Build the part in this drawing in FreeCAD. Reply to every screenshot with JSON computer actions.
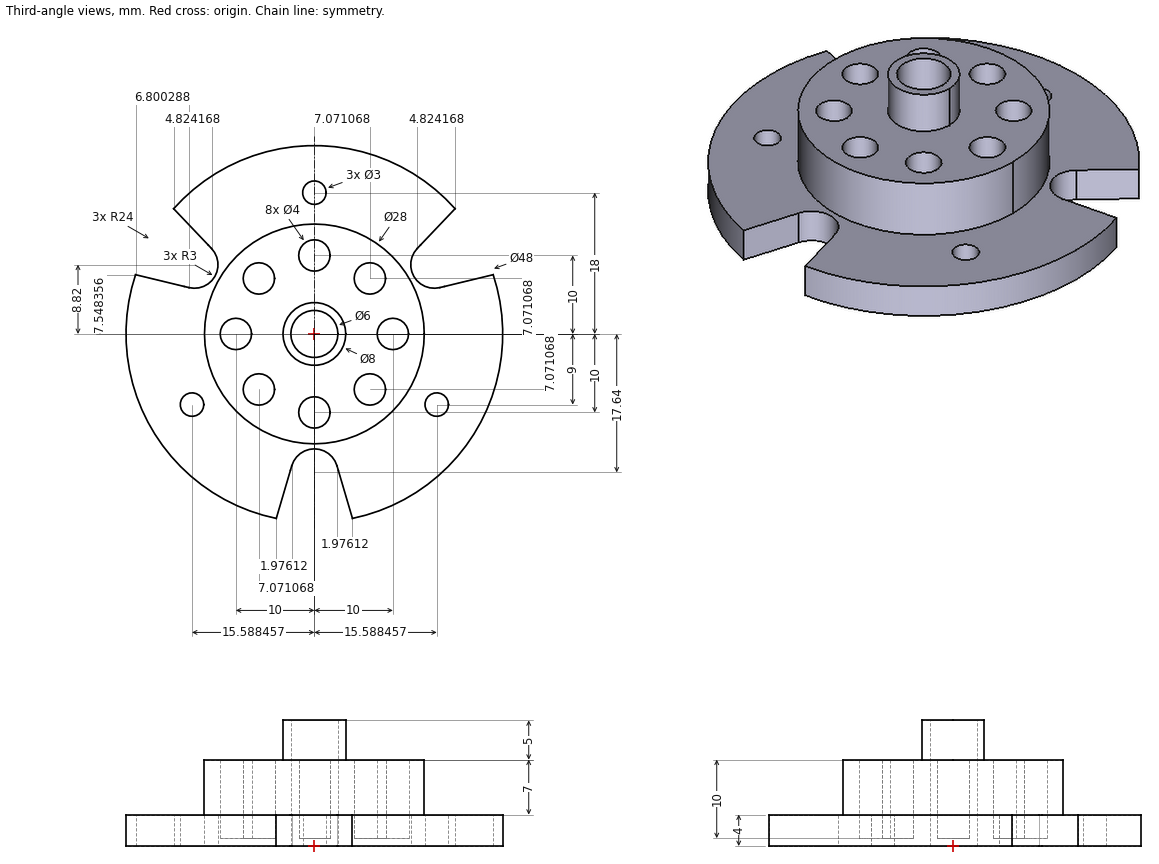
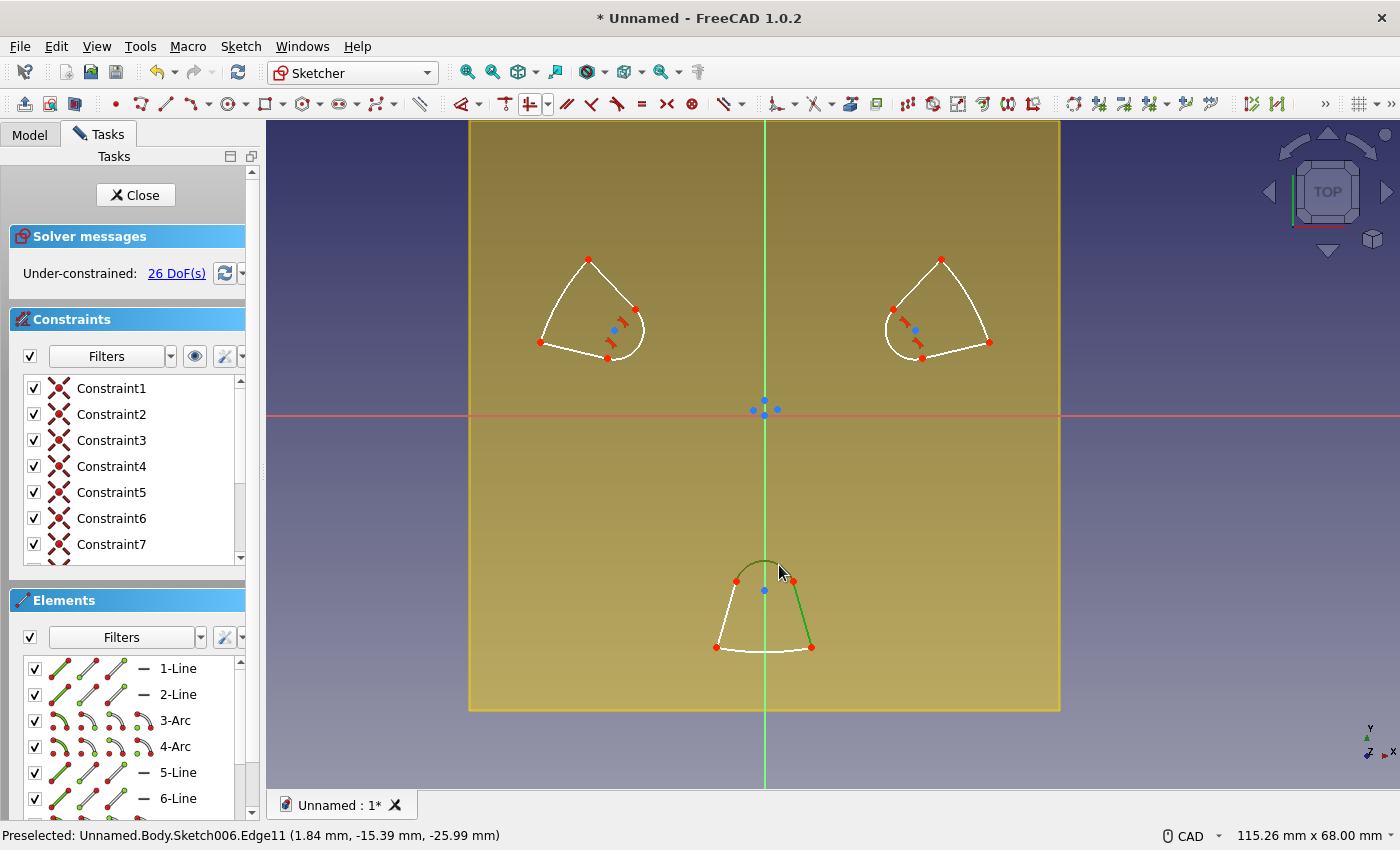
{"action": "key", "text": "t"}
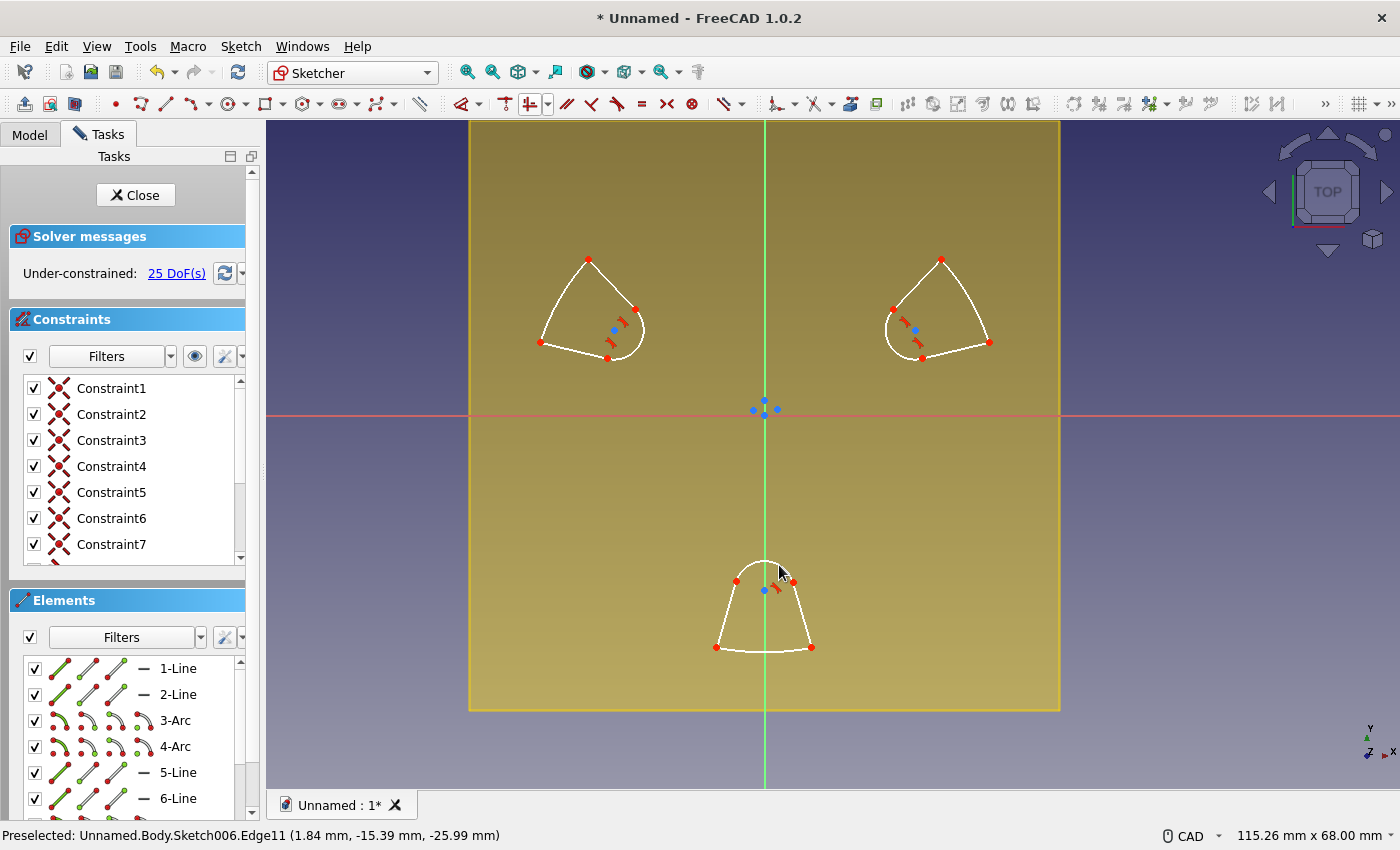
{"action": "left_click", "coordinate": [730, 602]}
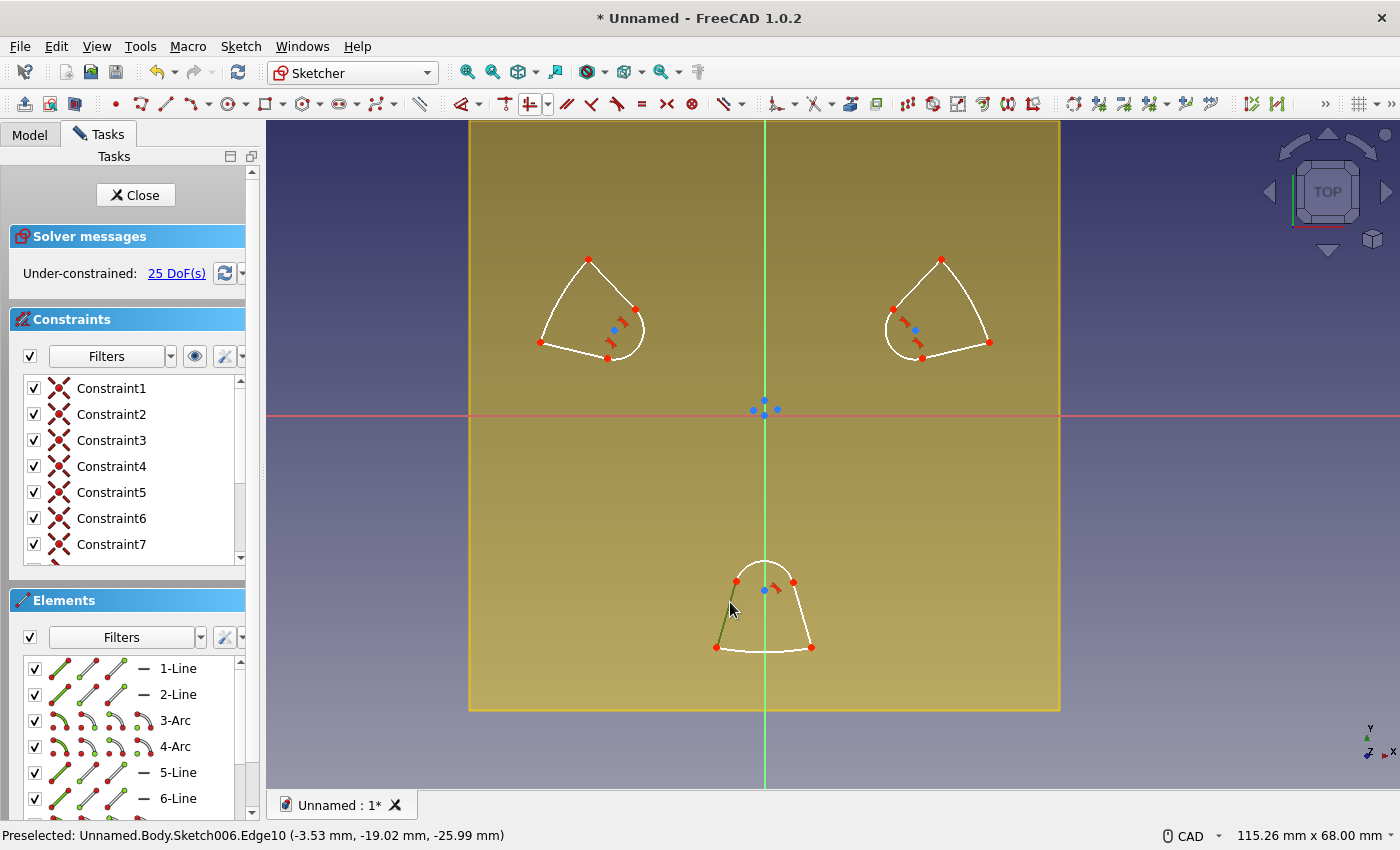
{"action": "left_click", "coordinate": [779, 565]}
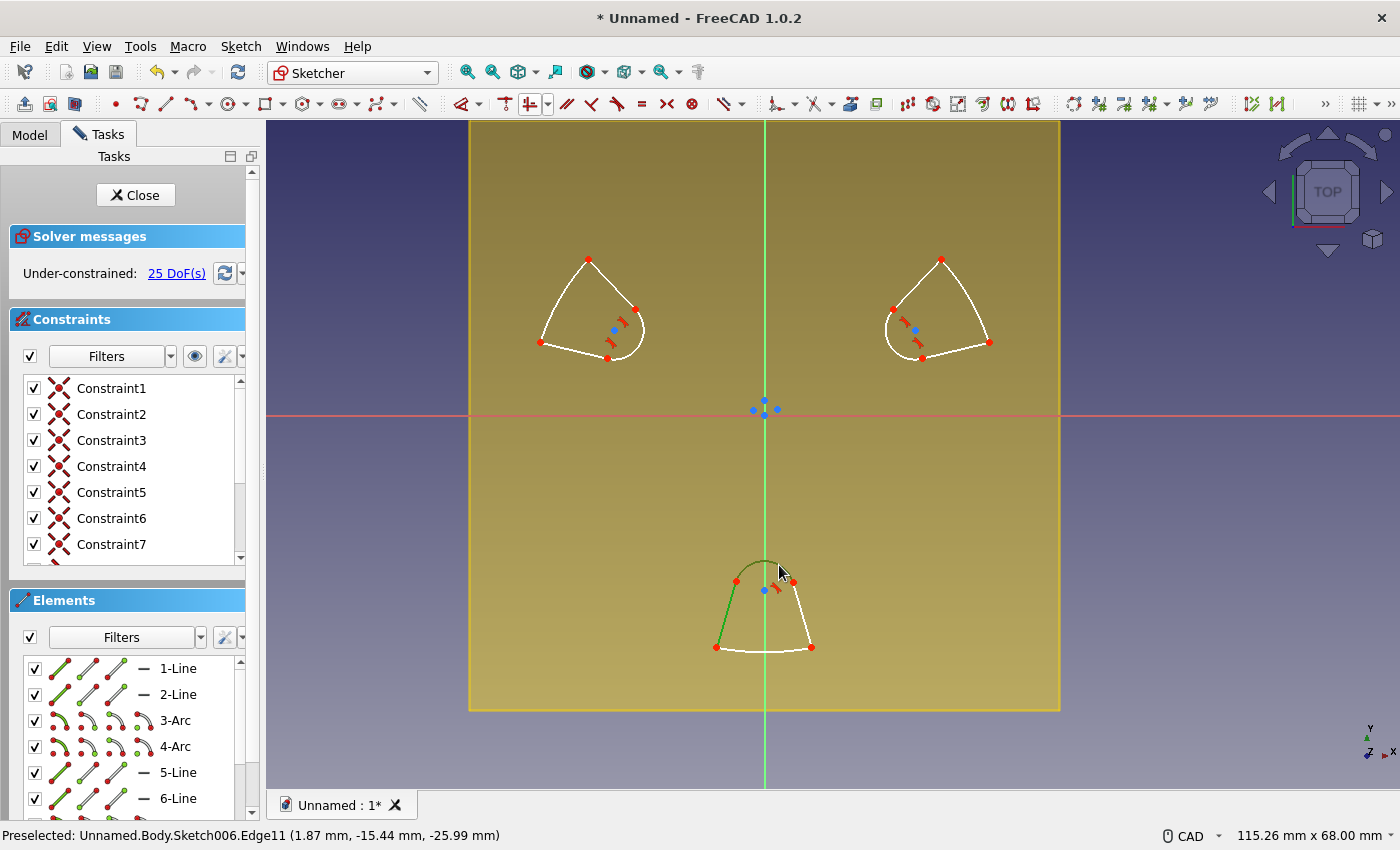
{"action": "key", "text": "t"}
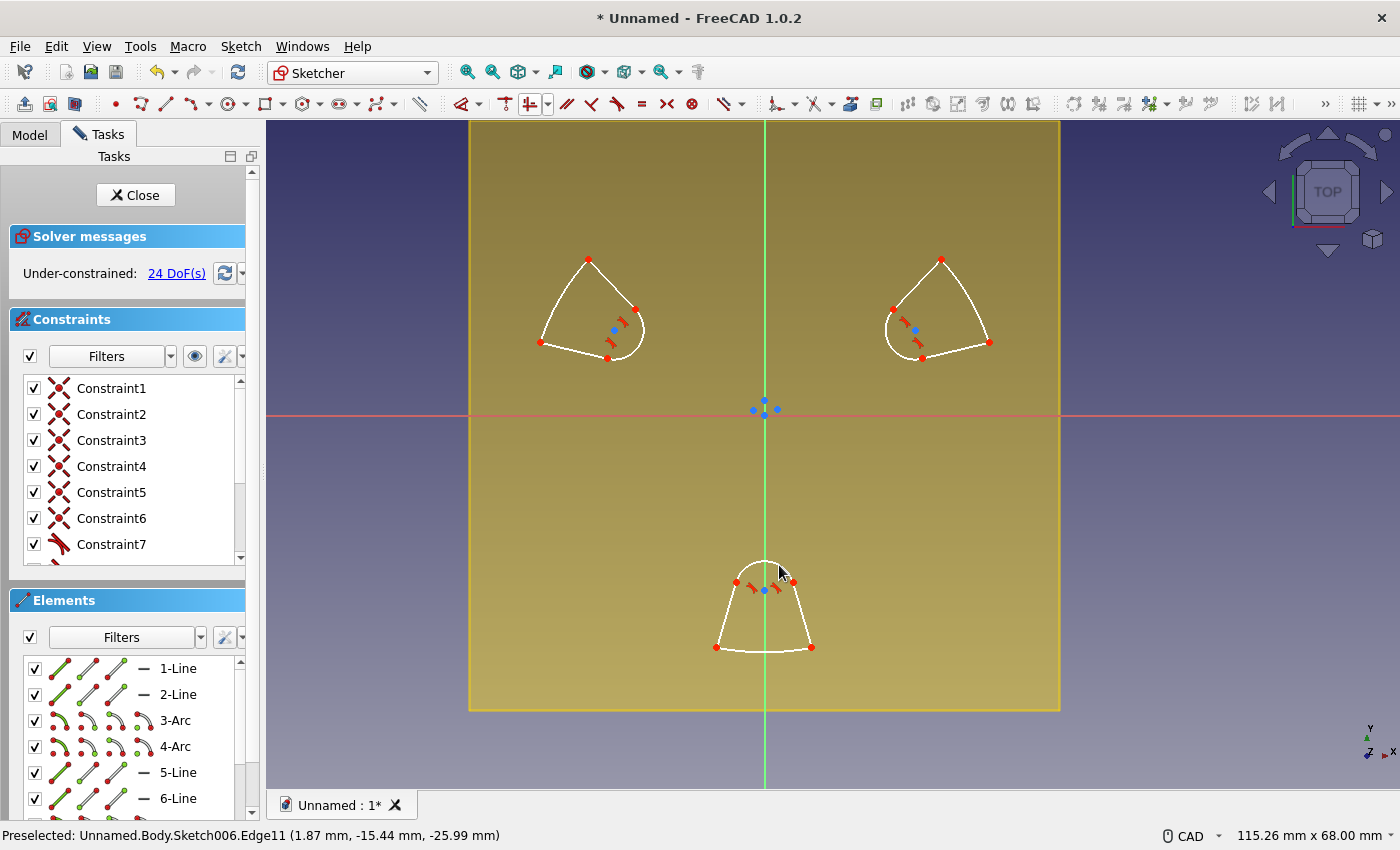
{"action": "left_click", "coordinate": [570, 282]}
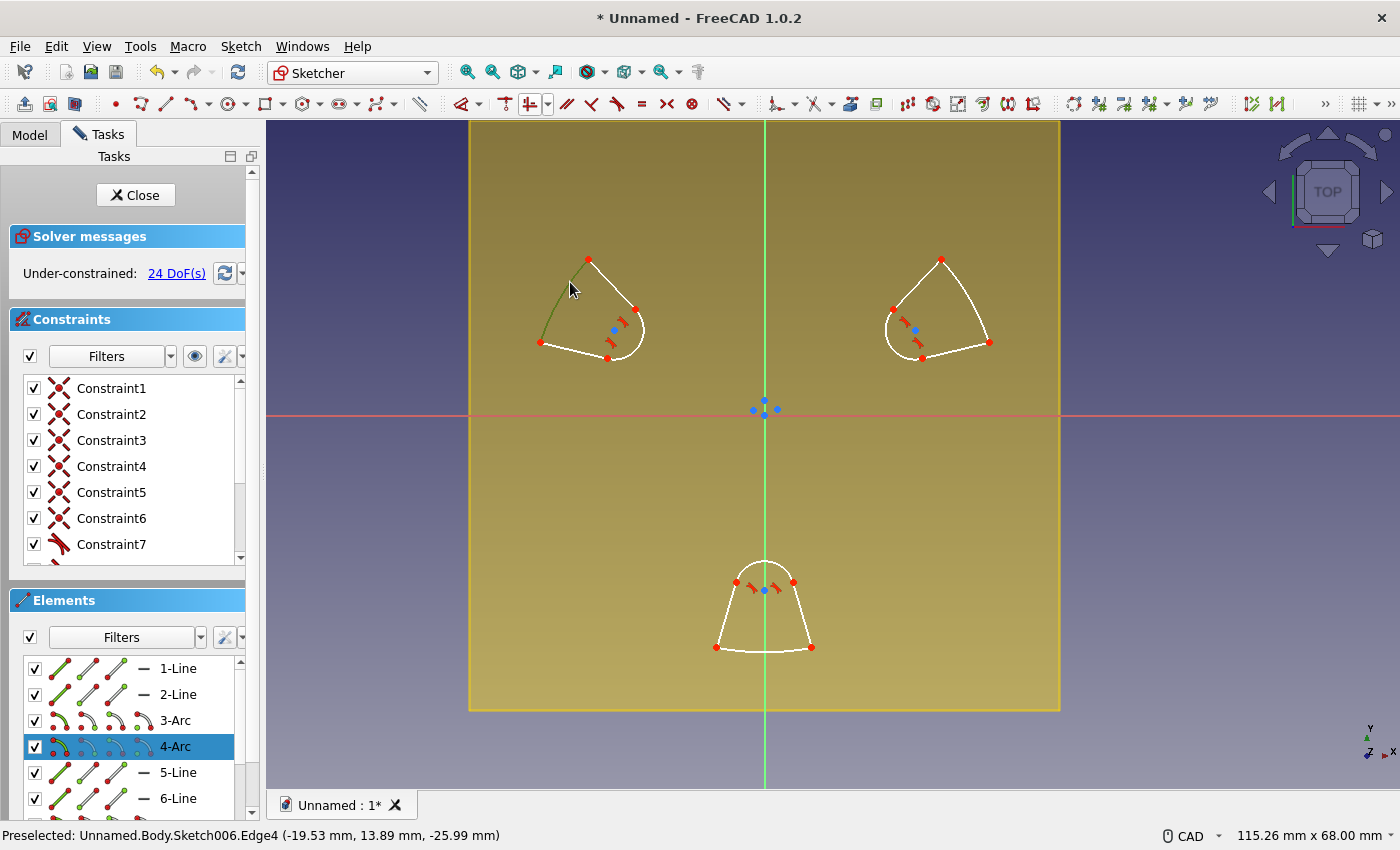
{"action": "left_click", "coordinate": [978, 316]}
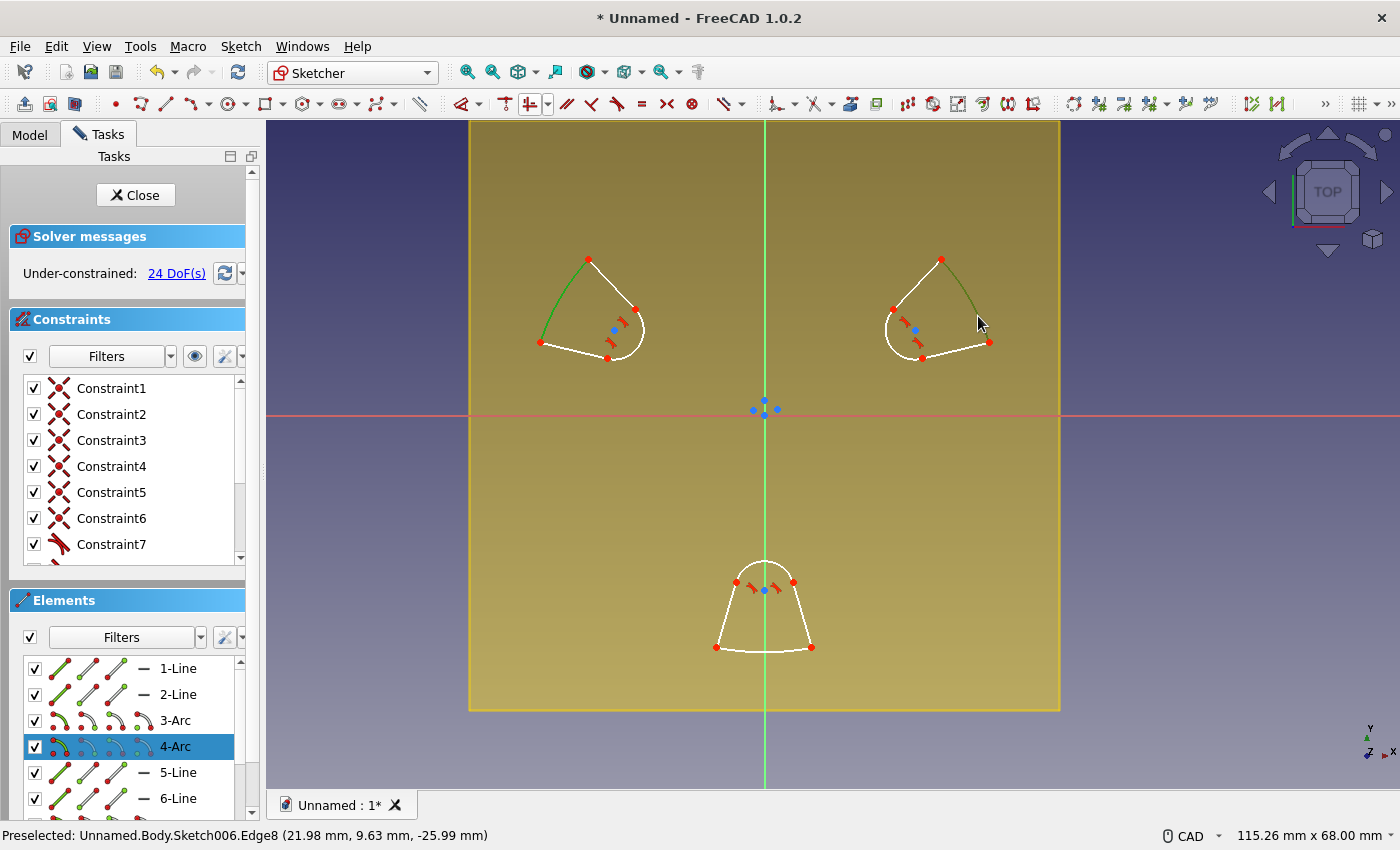
{"action": "key", "text": "c"}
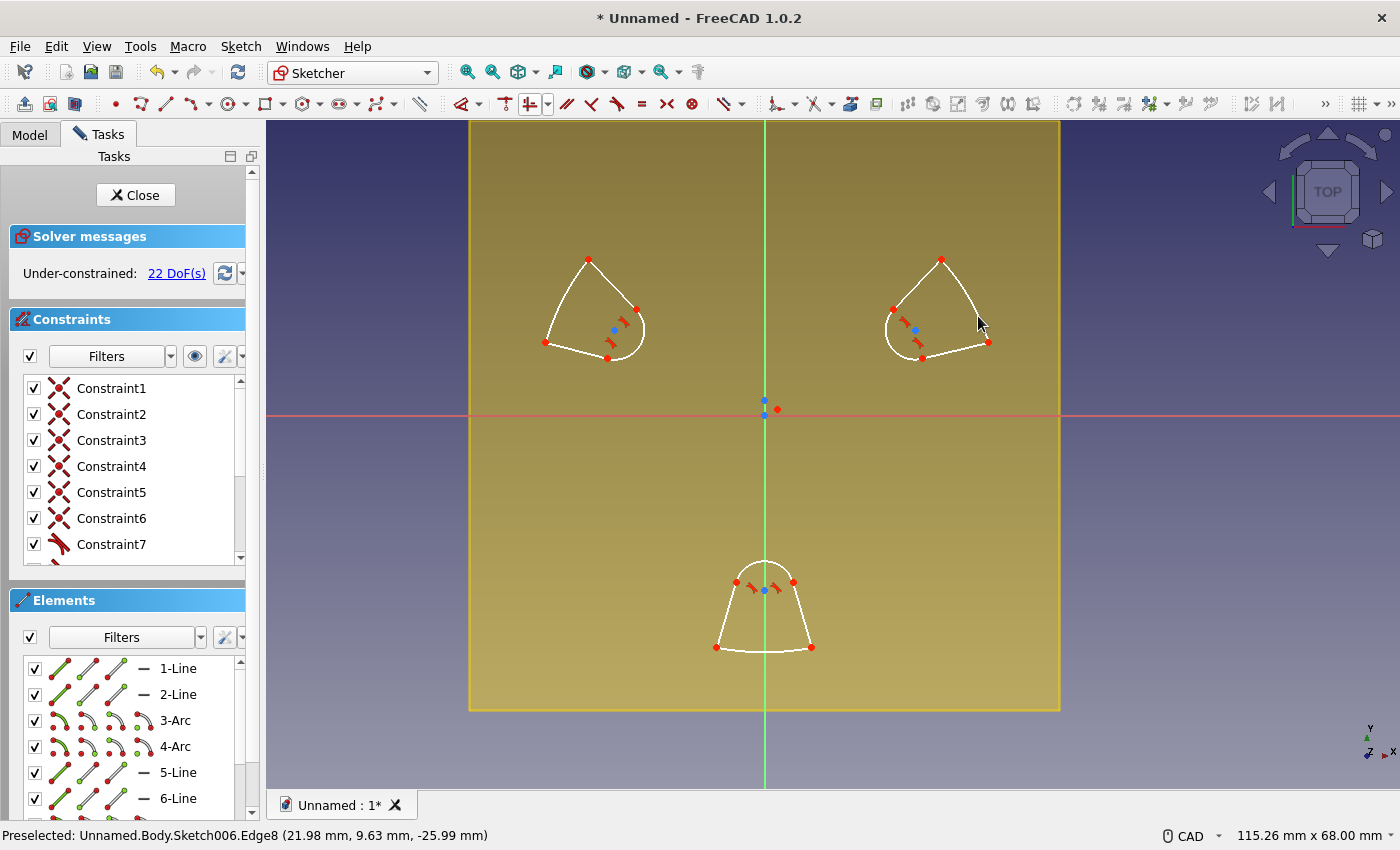
{"action": "left_click", "coordinate": [572, 283]}